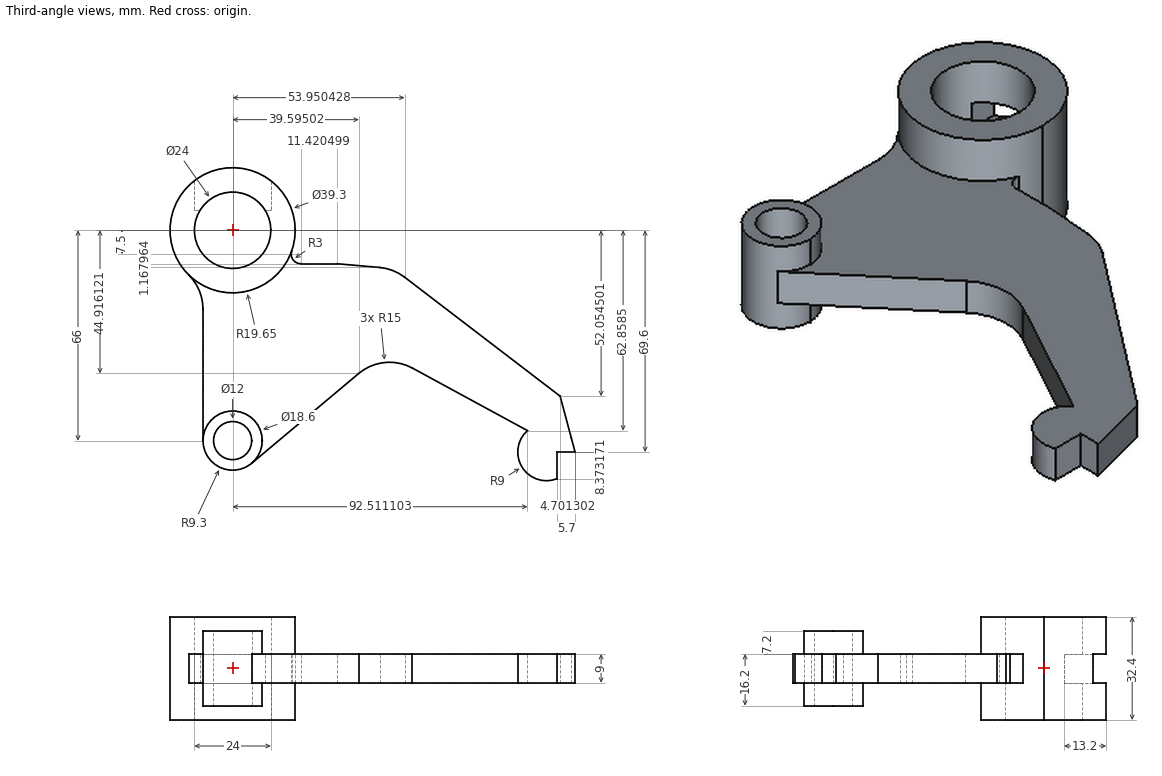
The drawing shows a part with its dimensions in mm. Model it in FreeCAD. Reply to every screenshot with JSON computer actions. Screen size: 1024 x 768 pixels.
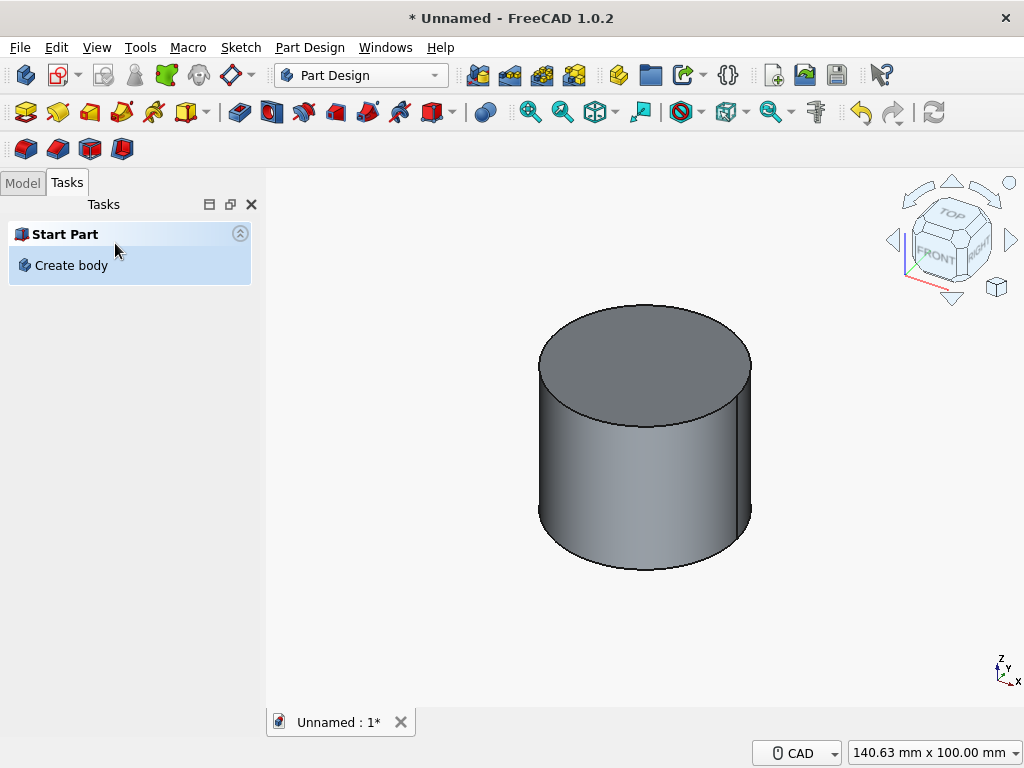
{"action": "left_click", "coordinate": [58, 76]}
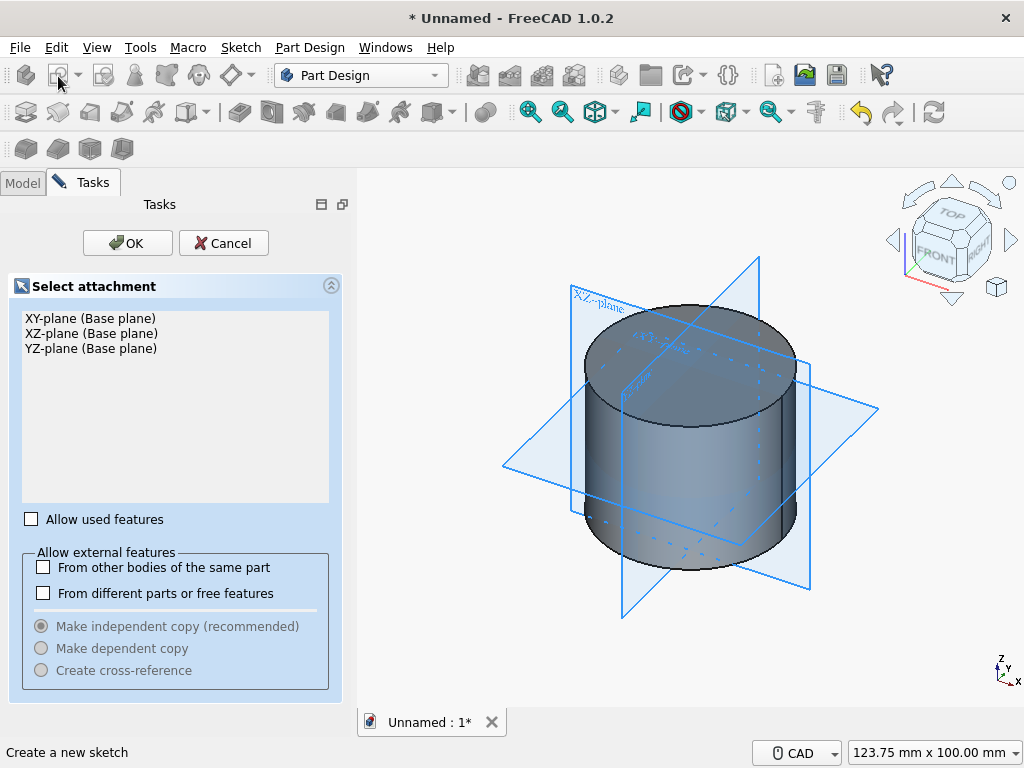
{"action": "left_click", "coordinate": [82, 318]}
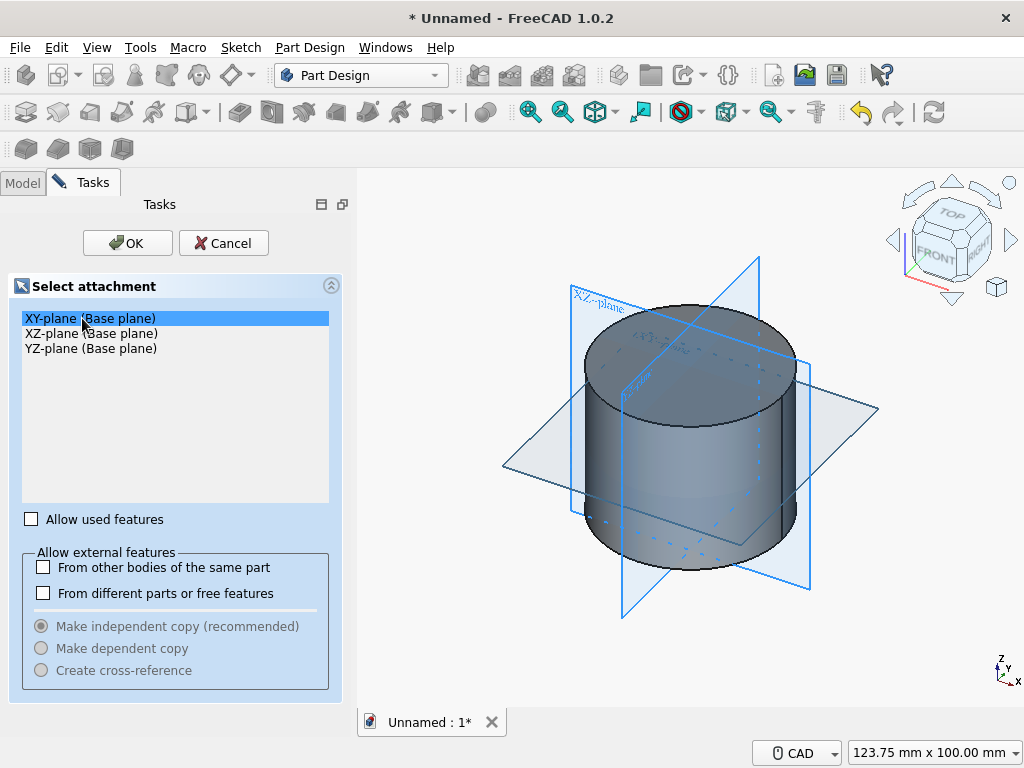
{"action": "left_click", "coordinate": [128, 243]}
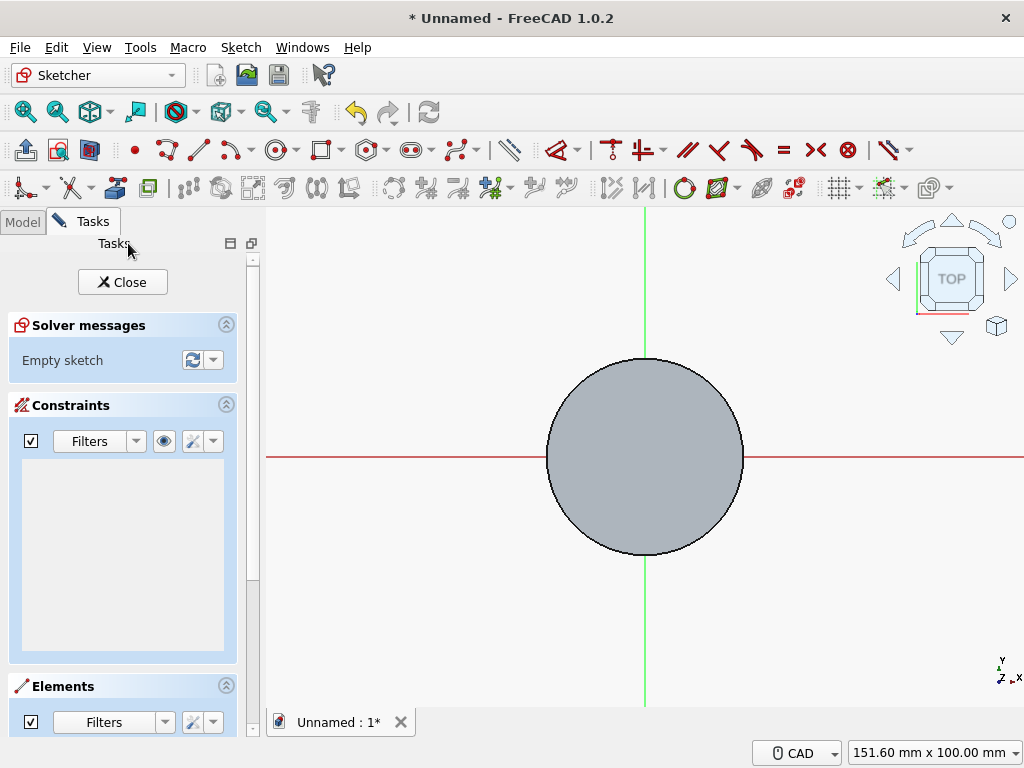
{"action": "key", "text": "q s"}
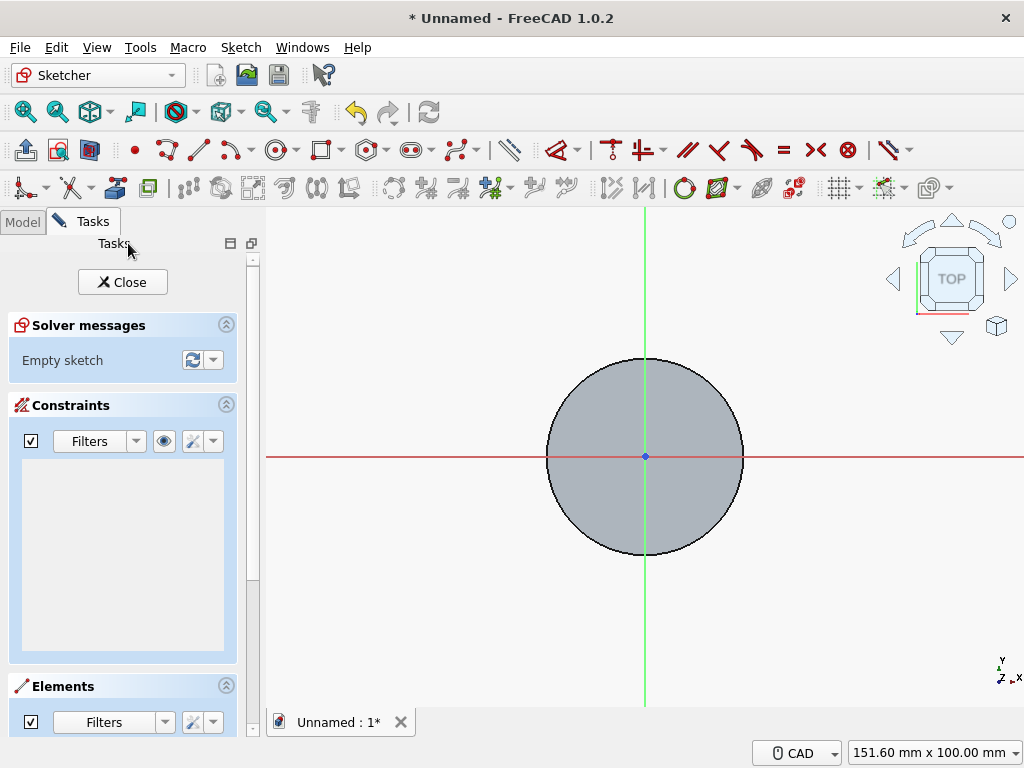
{"action": "scroll", "coordinate": [294, 235], "scroll_direction": "down", "scroll_amount": 3}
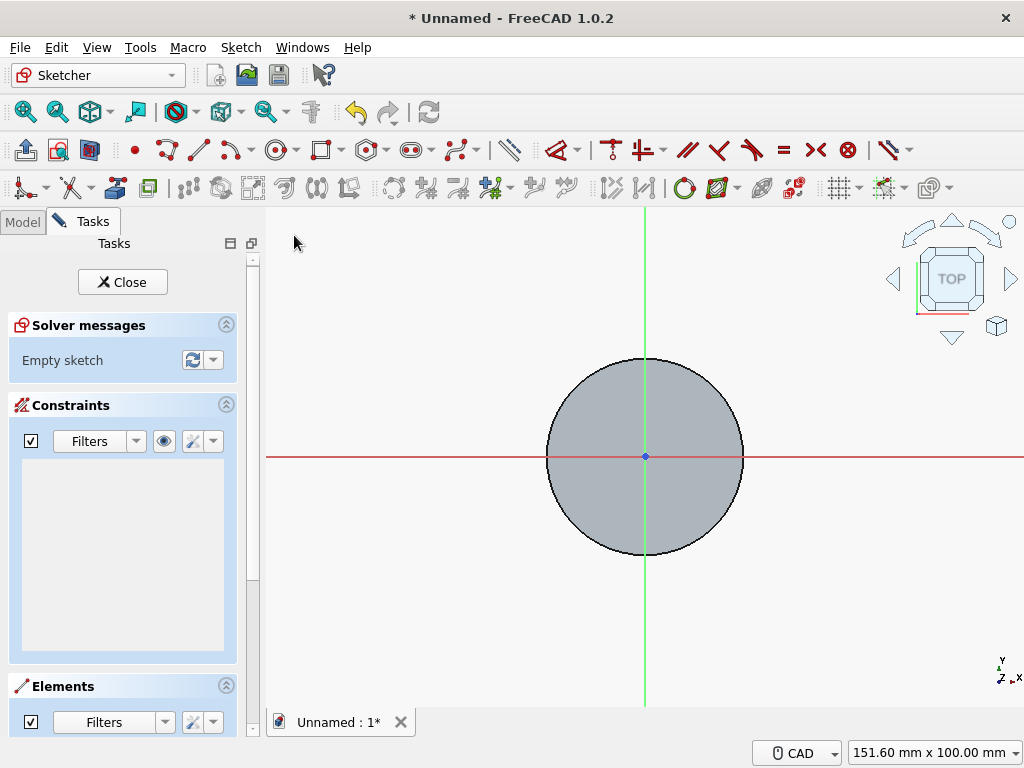
{"action": "key", "text": "g l"}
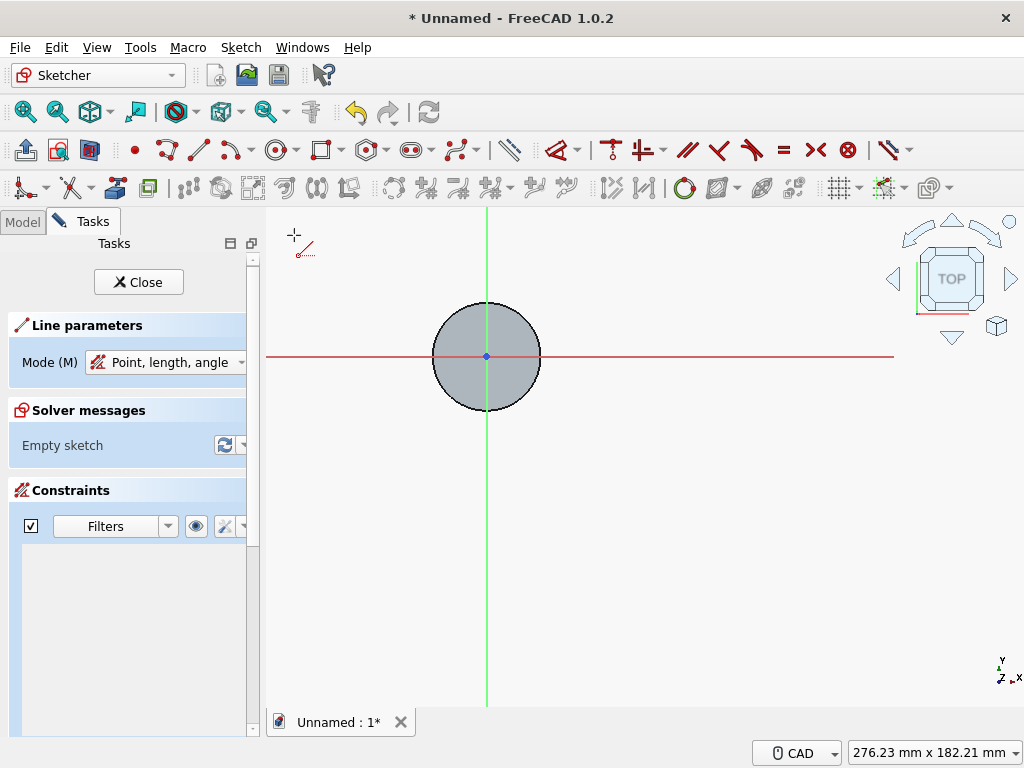
{"action": "left_click", "coordinate": [461, 425]}
{"action": "left_click", "coordinate": [461, 538]}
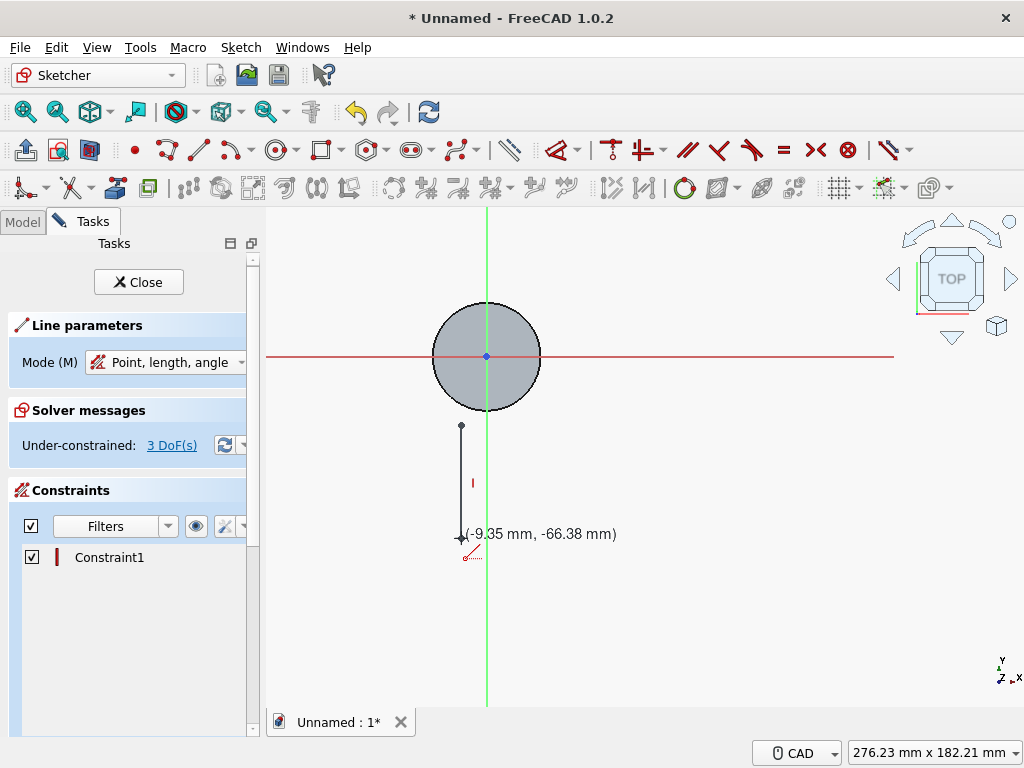
{"action": "left_click", "coordinate": [503, 558]}
{"action": "left_click", "coordinate": [595, 480]}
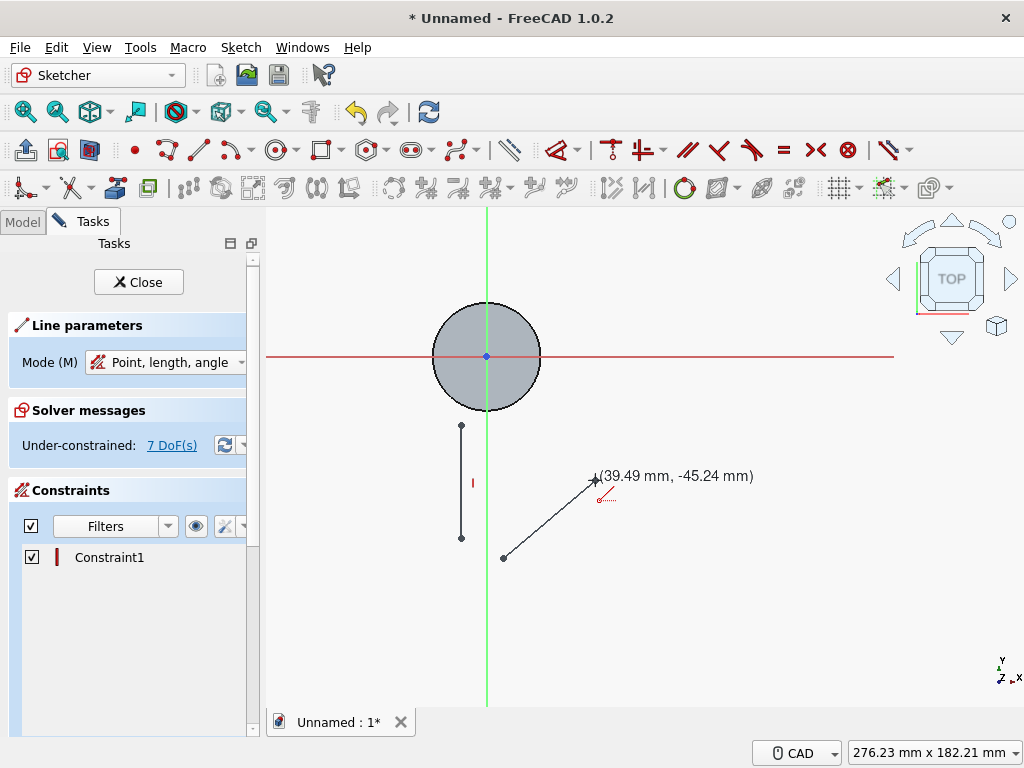
{"action": "left_click", "coordinate": [641, 475]}
{"action": "left_click", "coordinate": [741, 529]}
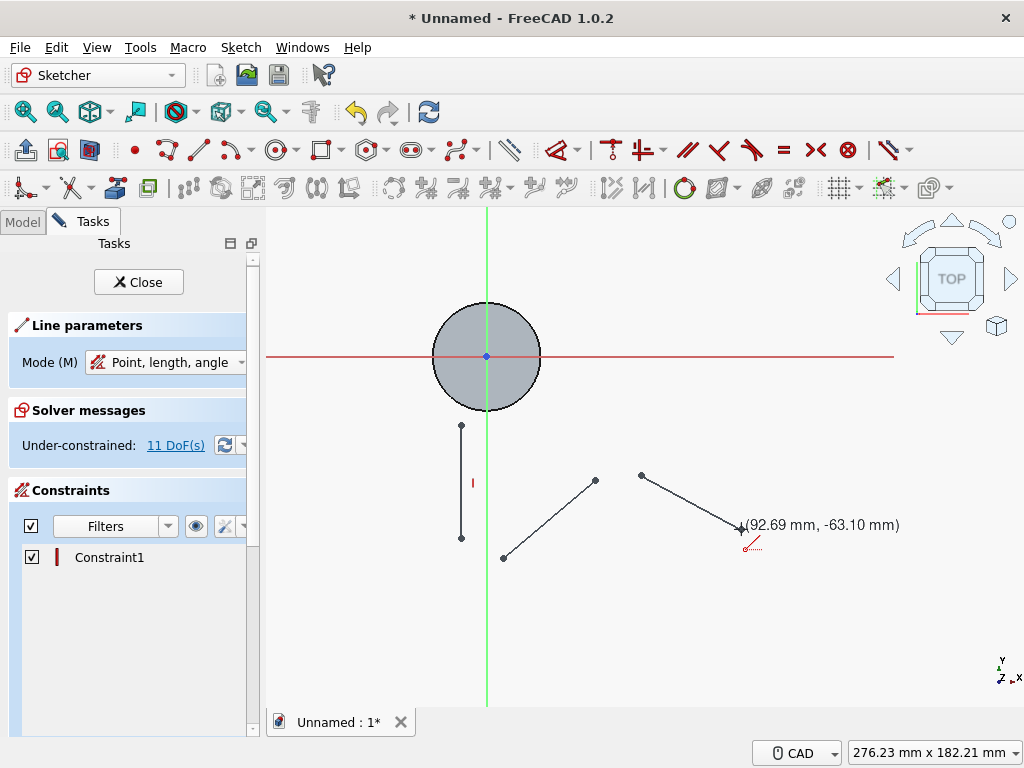
{"action": "key", "text": "g m"}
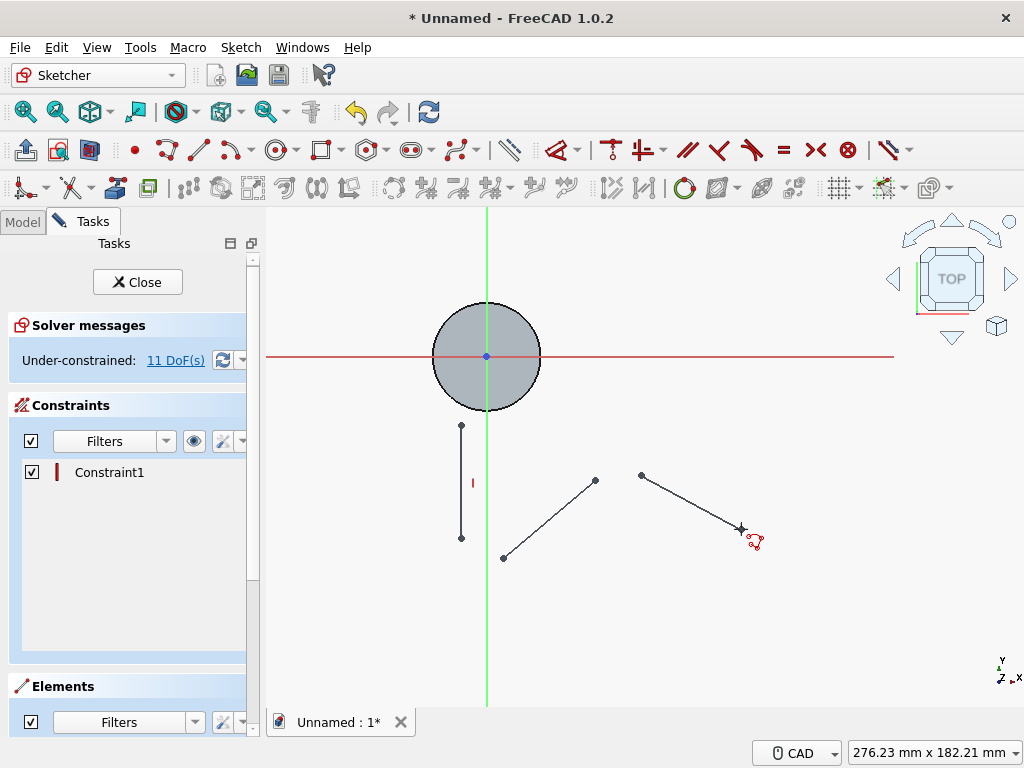
{"action": "left_click", "coordinate": [766, 571]}
{"action": "left_click", "coordinate": [766, 548]}
{"action": "left_click", "coordinate": [782, 548]}
{"action": "left_click", "coordinate": [769, 500]}
{"action": "left_click", "coordinate": [635, 397]}
{"action": "right_click", "coordinate": [635, 397]}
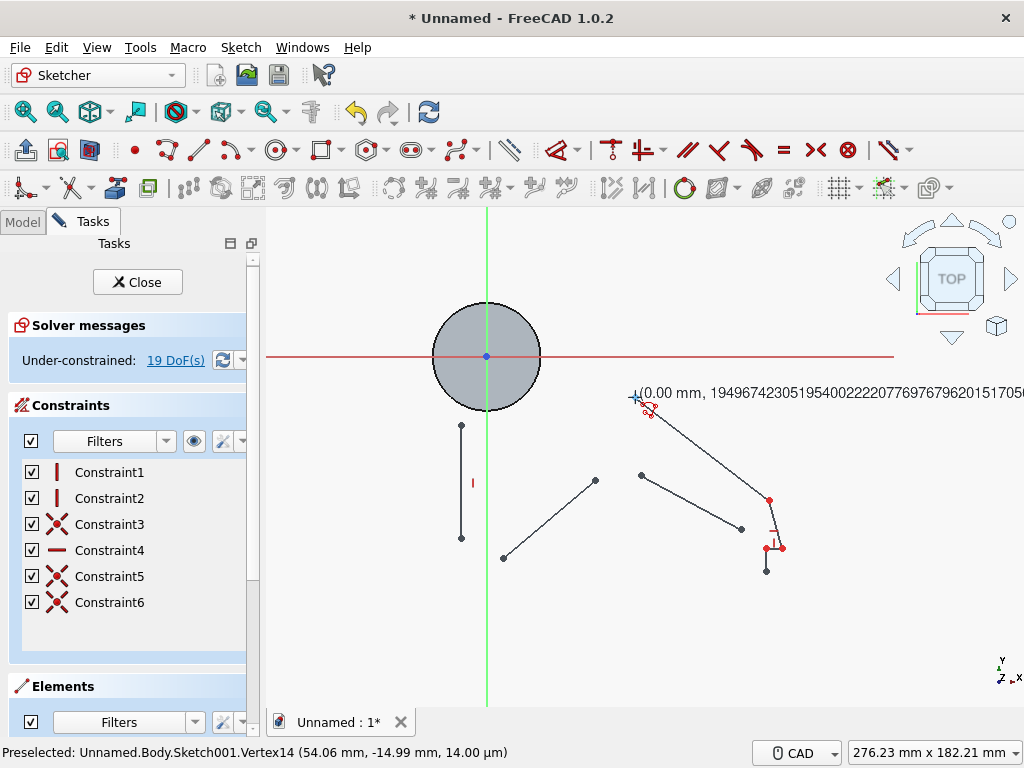
{"action": "left_click", "coordinate": [613, 389]}
{"action": "left_click", "coordinate": [577, 386]}
{"action": "left_click", "coordinate": [545, 386]}
{"action": "right_click", "coordinate": [545, 386]}